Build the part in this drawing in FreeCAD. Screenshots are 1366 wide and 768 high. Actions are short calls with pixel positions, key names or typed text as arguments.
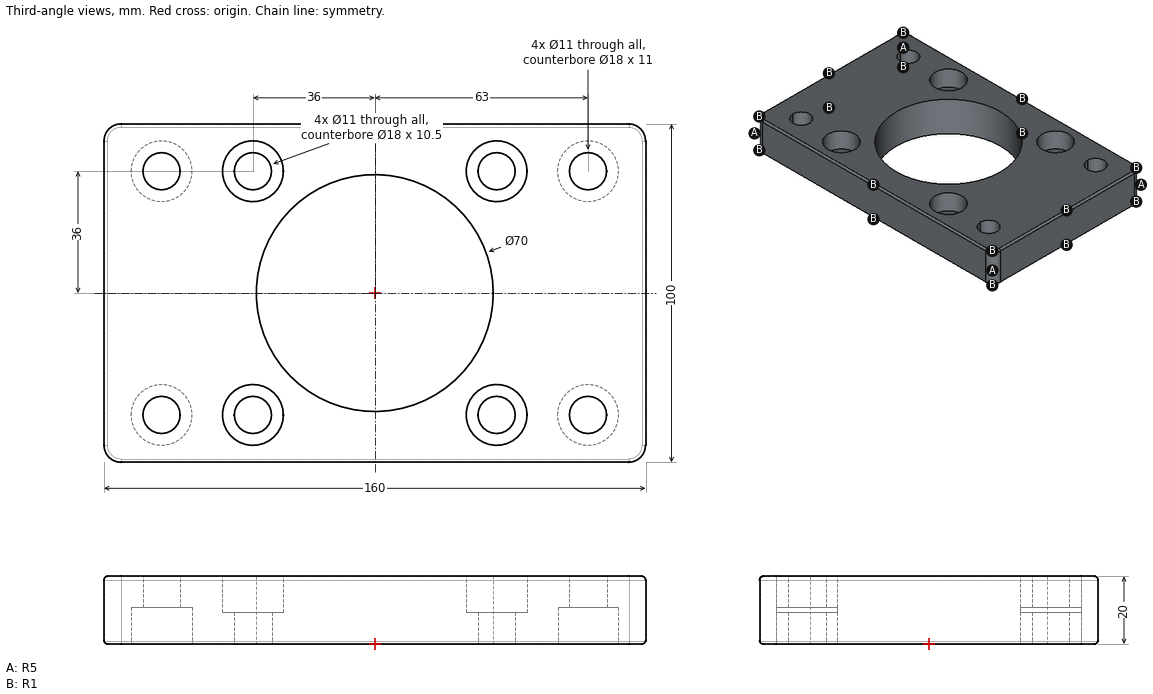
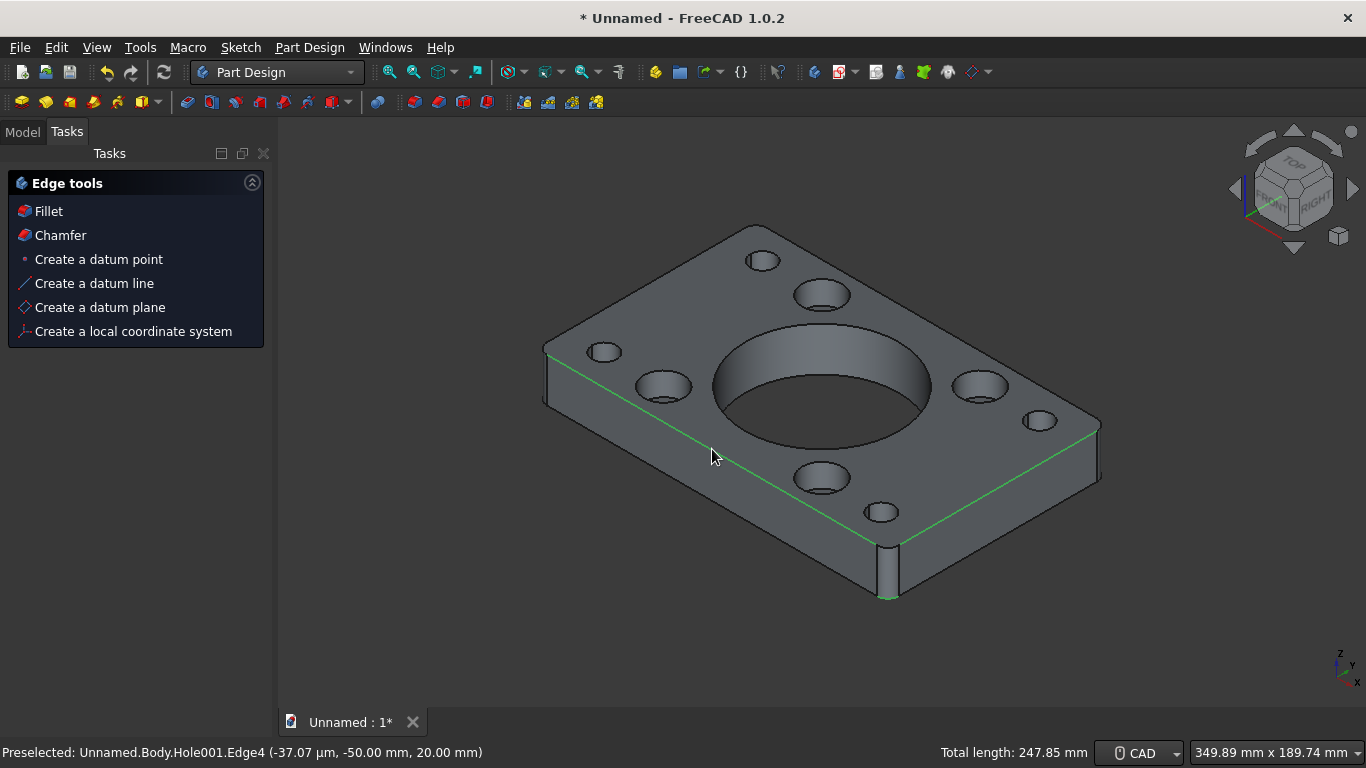
click(1101, 424, ctrl)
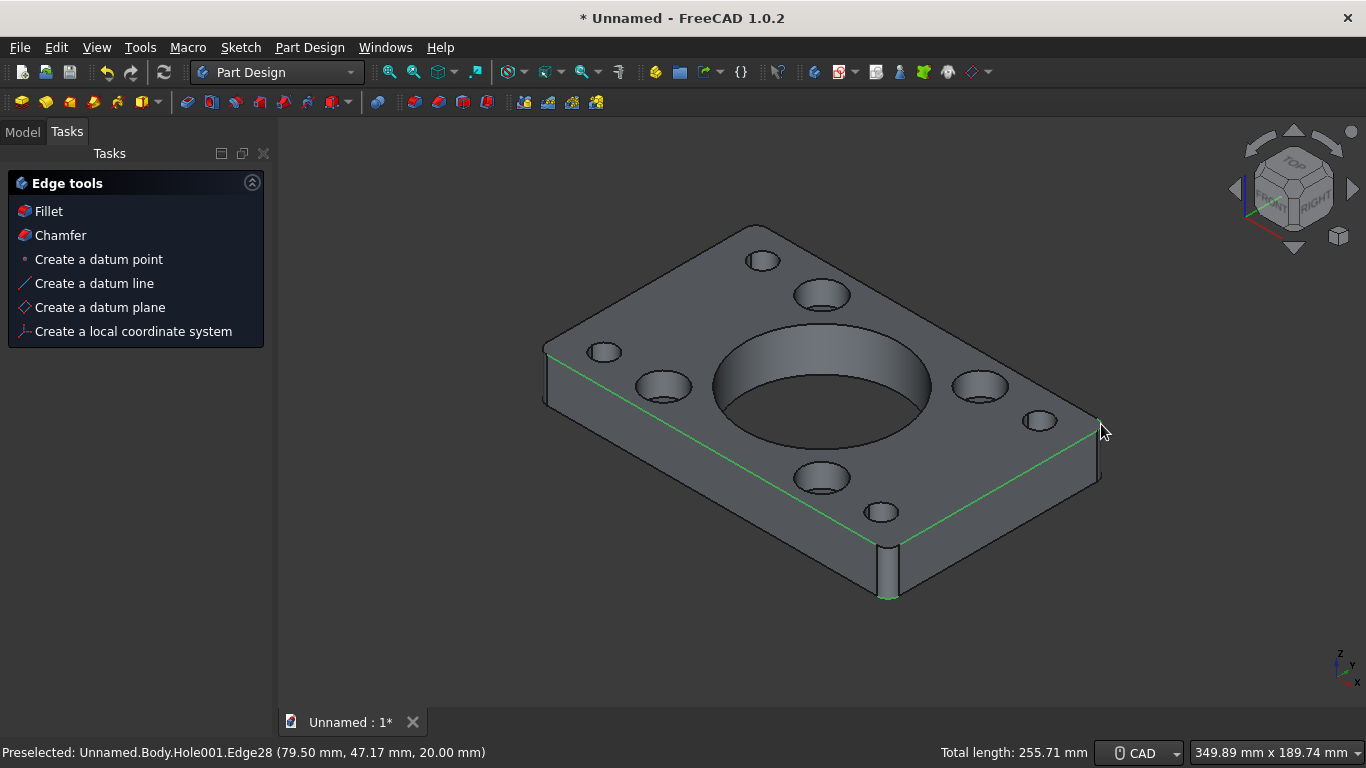
click(543, 348, ctrl)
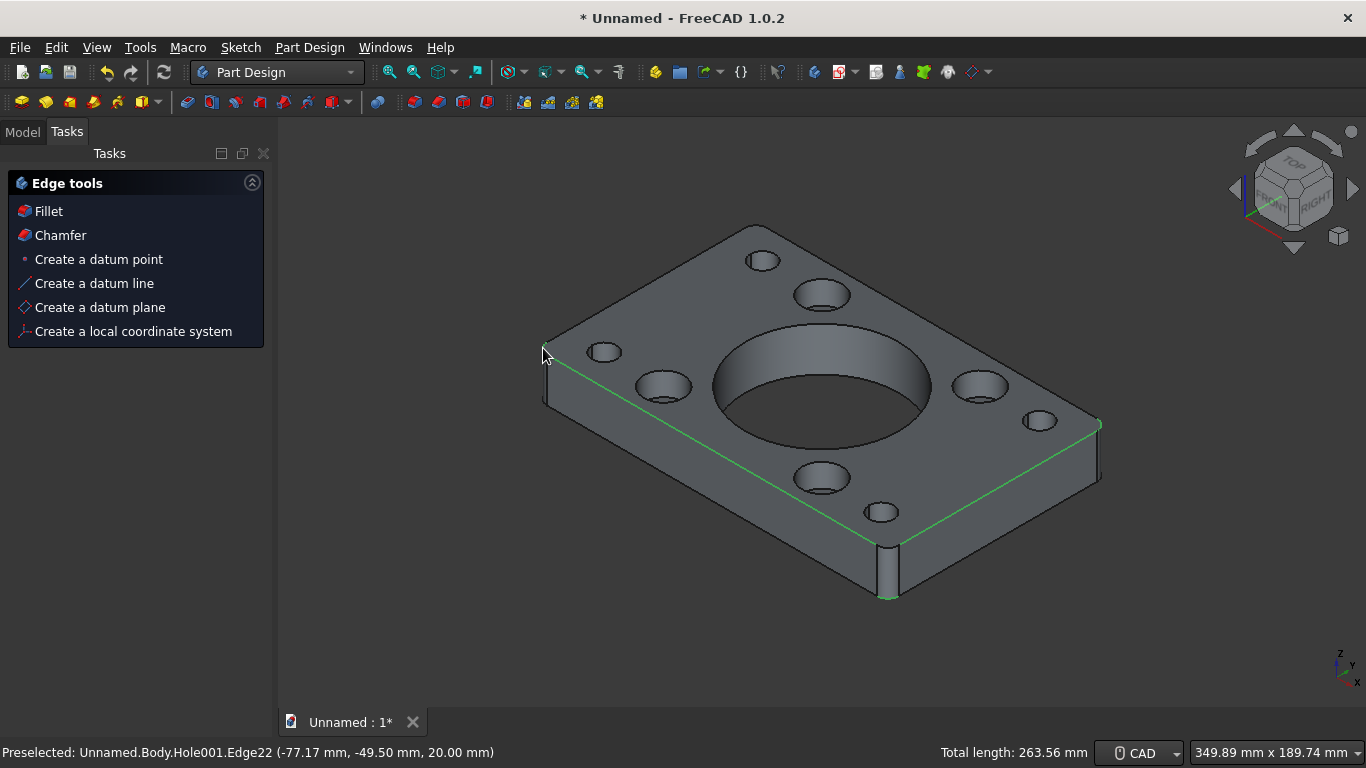
click(888, 547, ctrl)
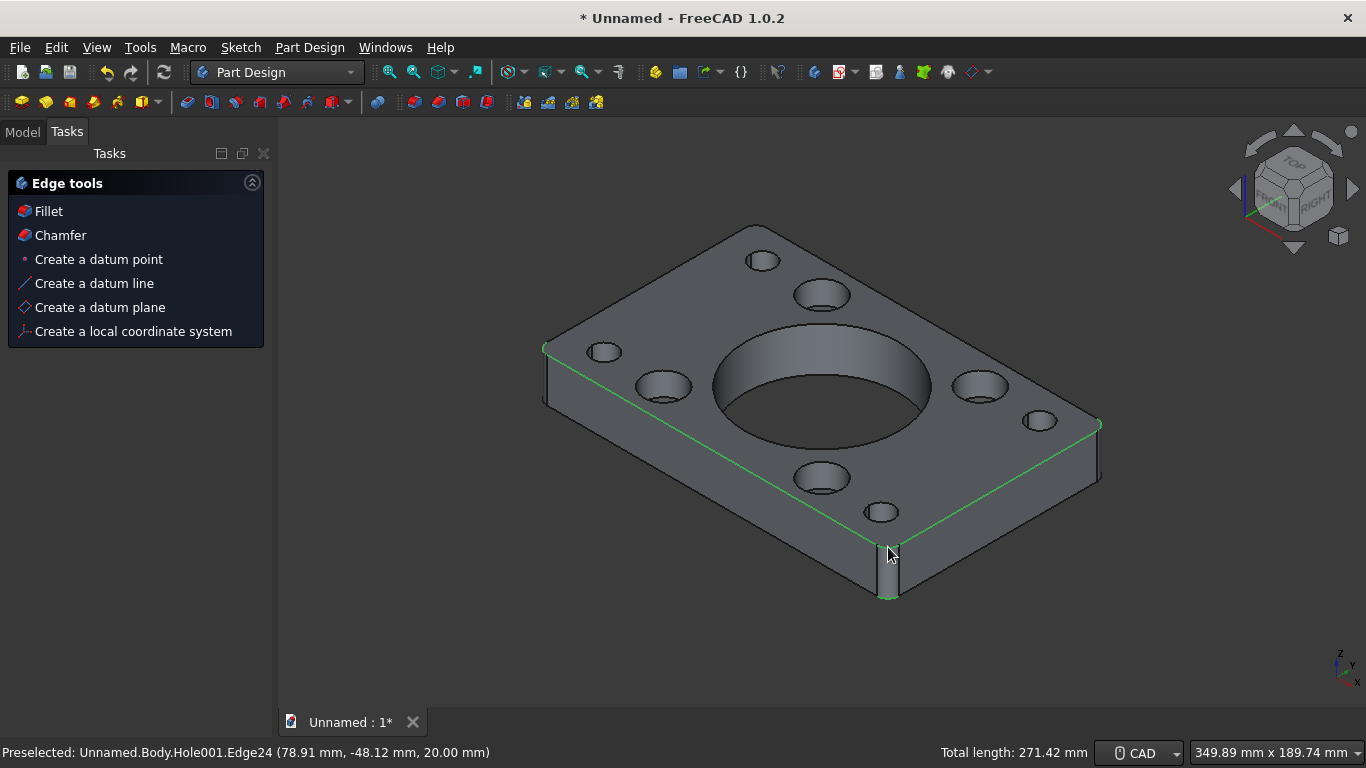
key(2)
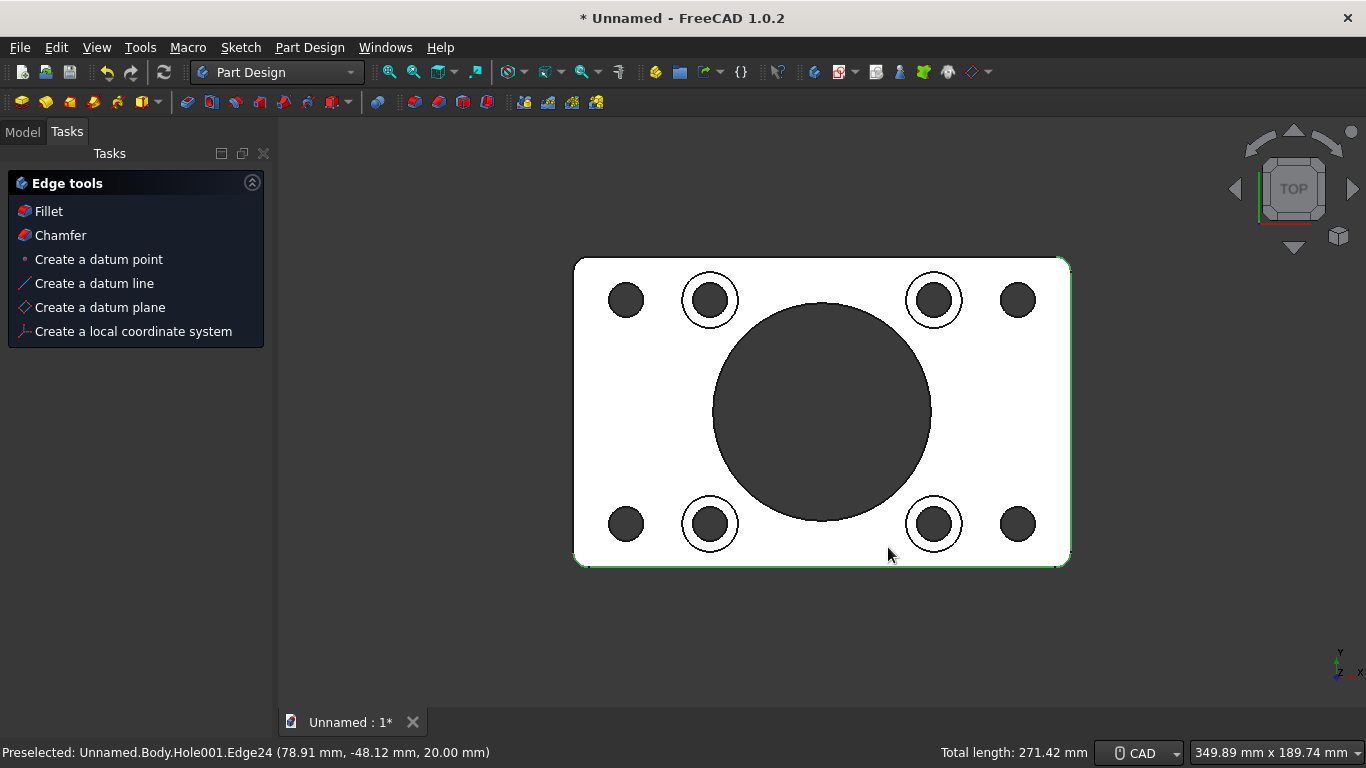
click(573, 411, ctrl)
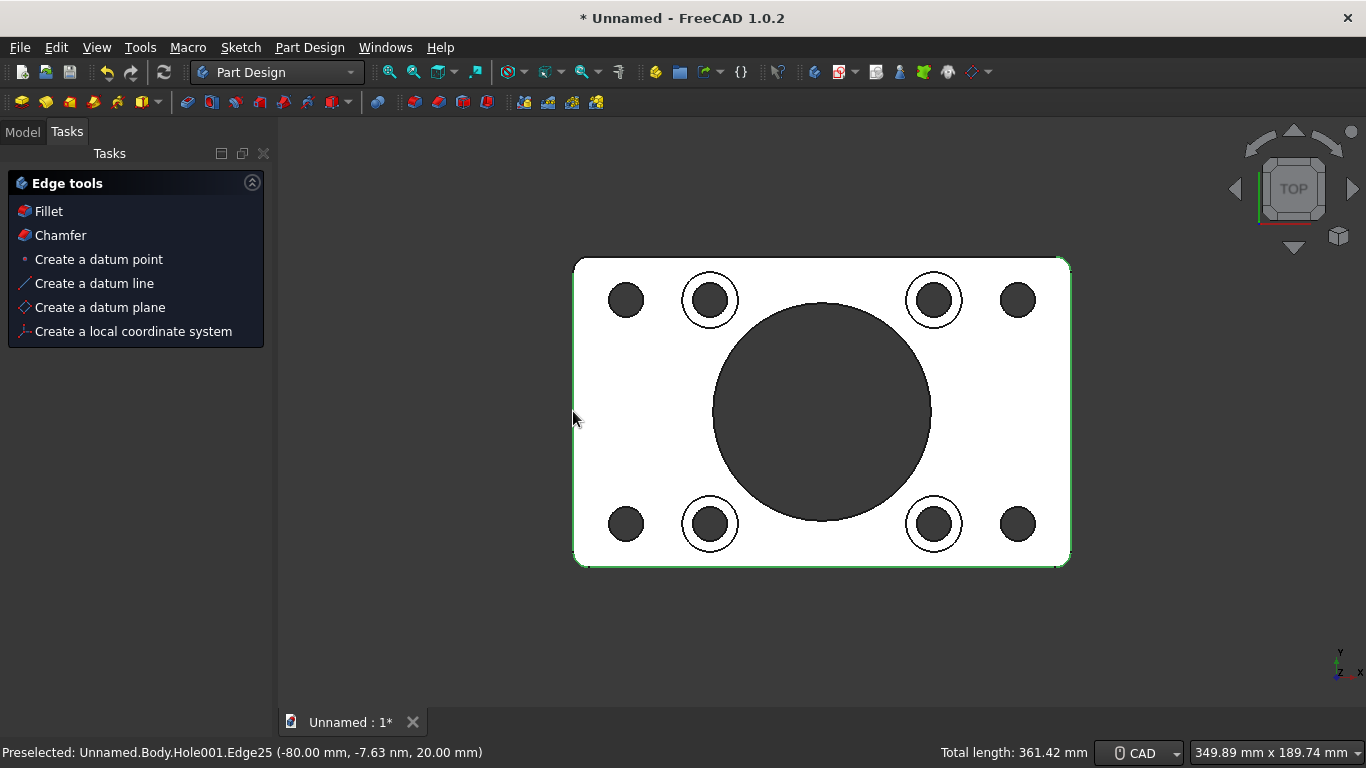
click(822, 256, ctrl)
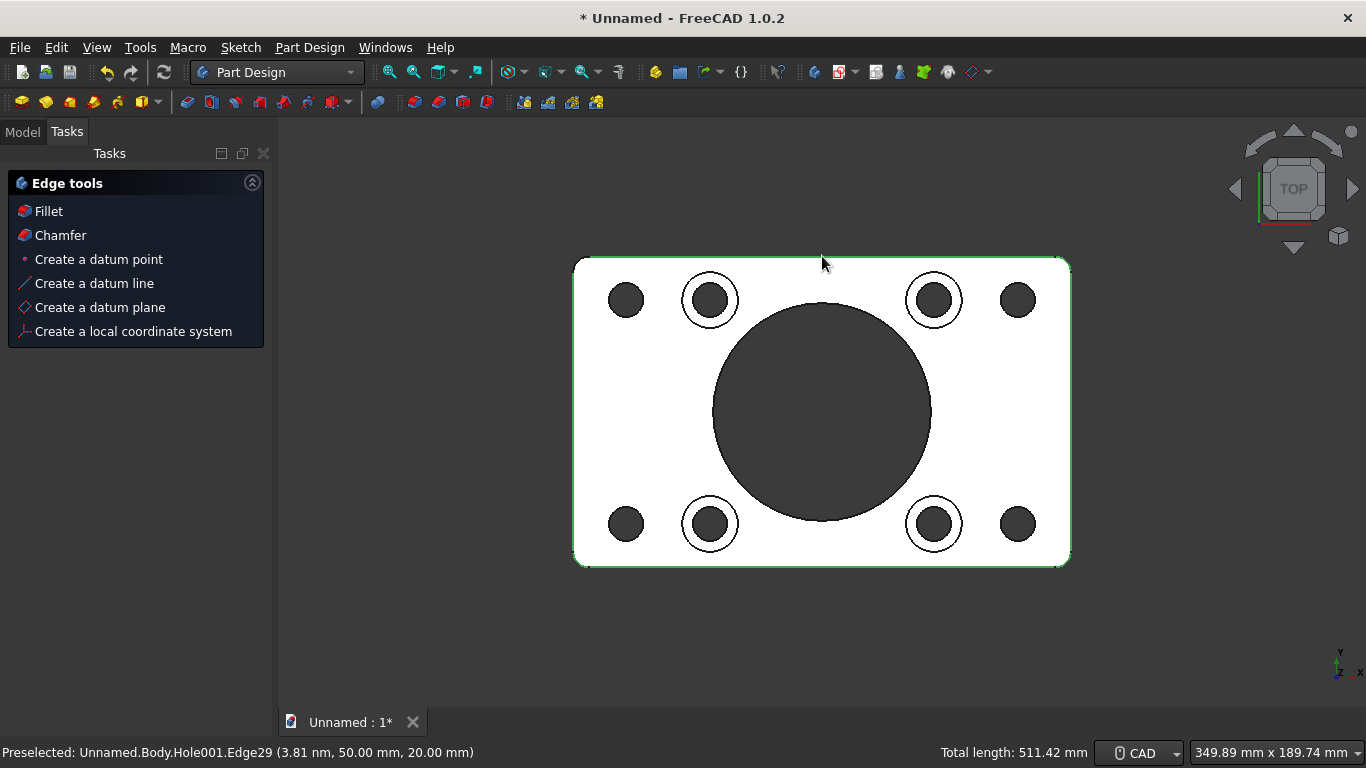
click(578, 260, ctrl)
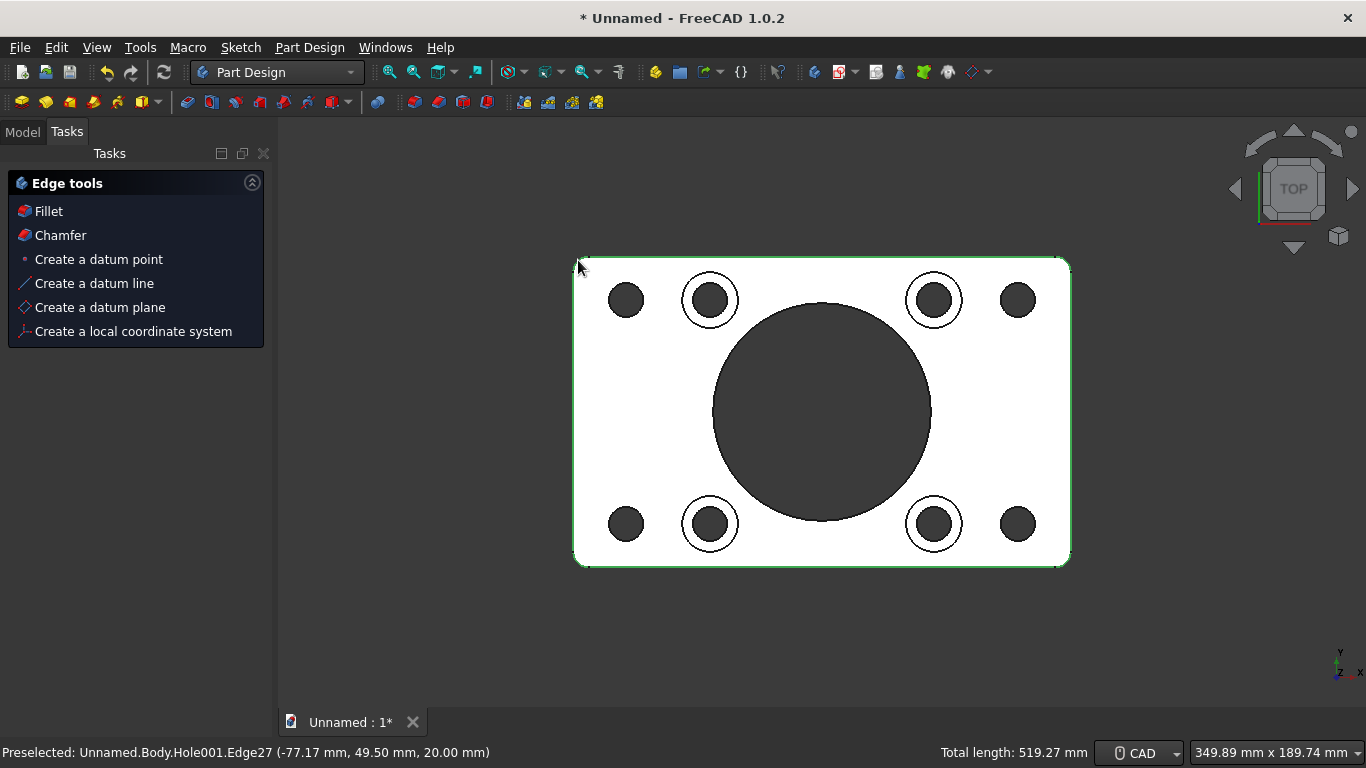
key(0)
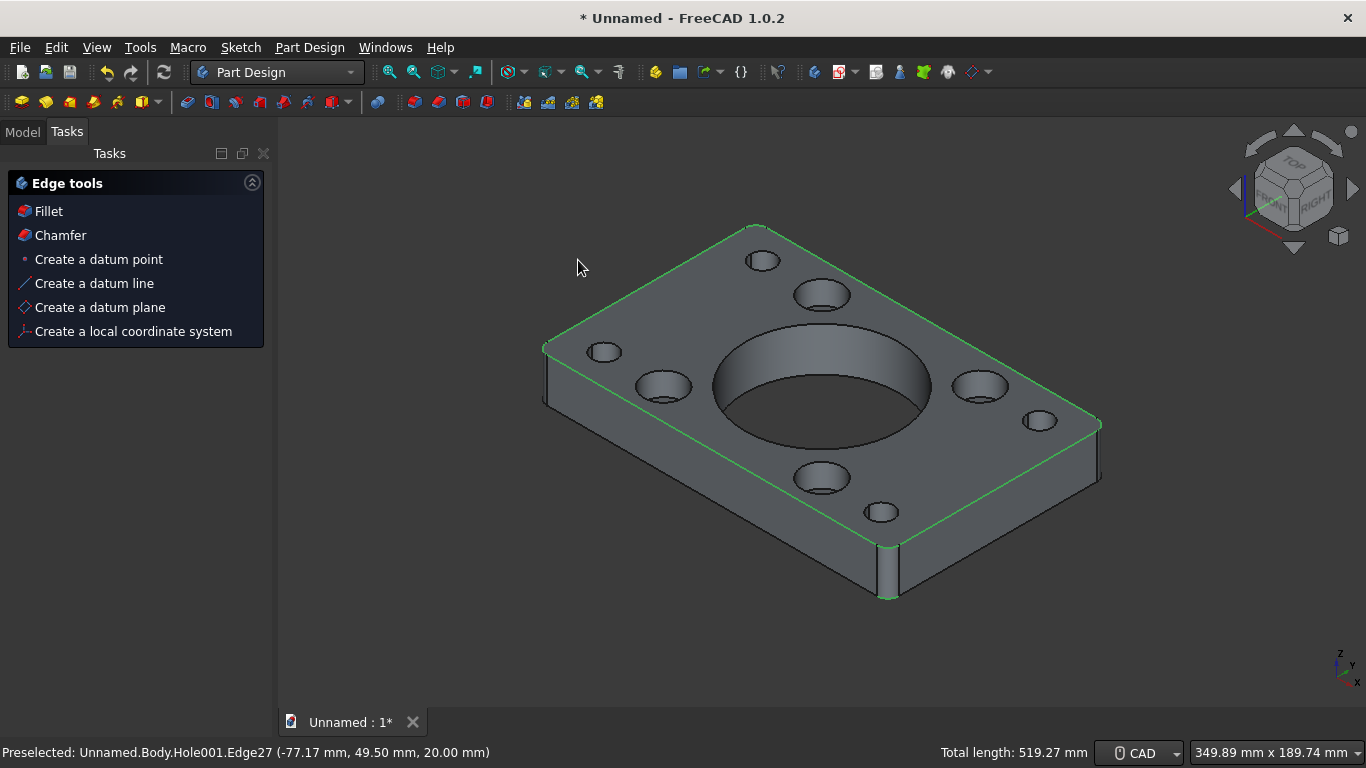
key(1)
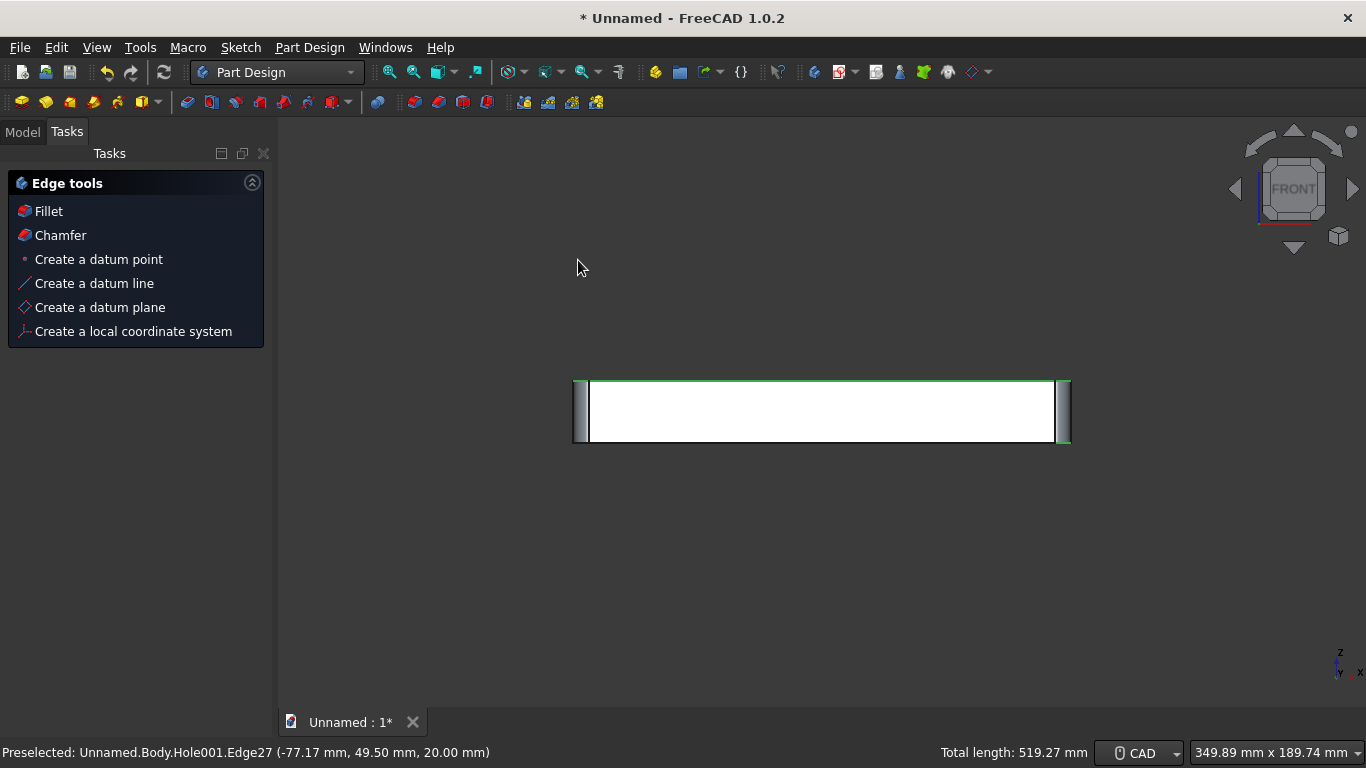
click(822, 442, ctrl)